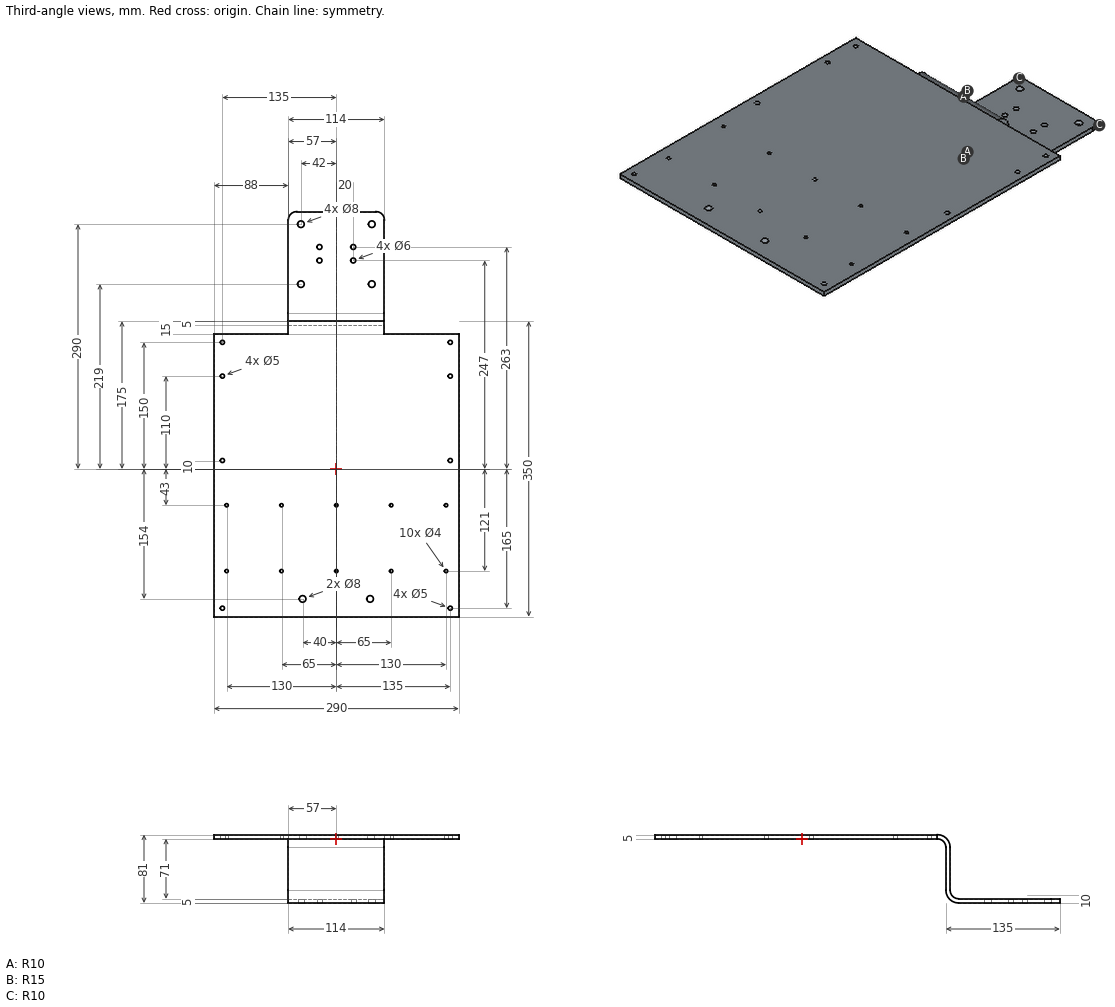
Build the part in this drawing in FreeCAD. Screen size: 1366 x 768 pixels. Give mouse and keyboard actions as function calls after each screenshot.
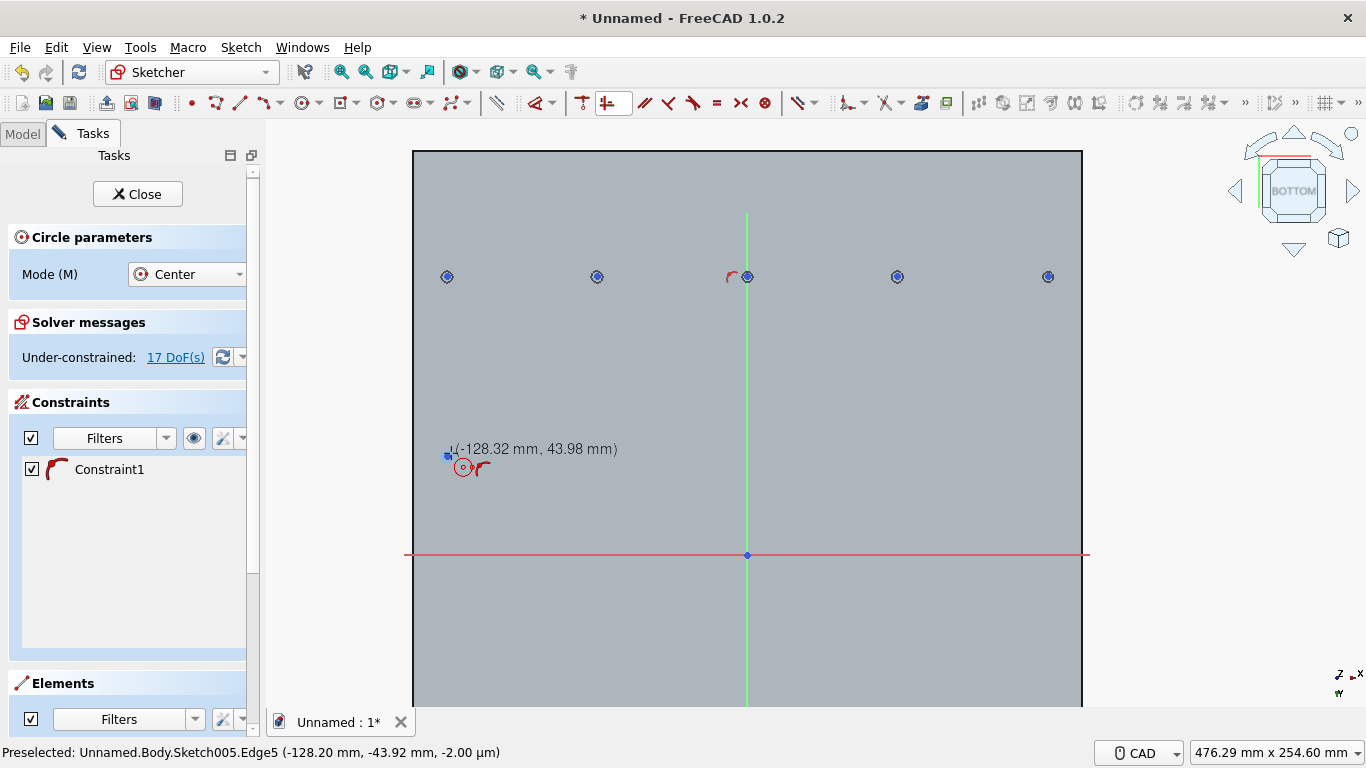
click(597, 456)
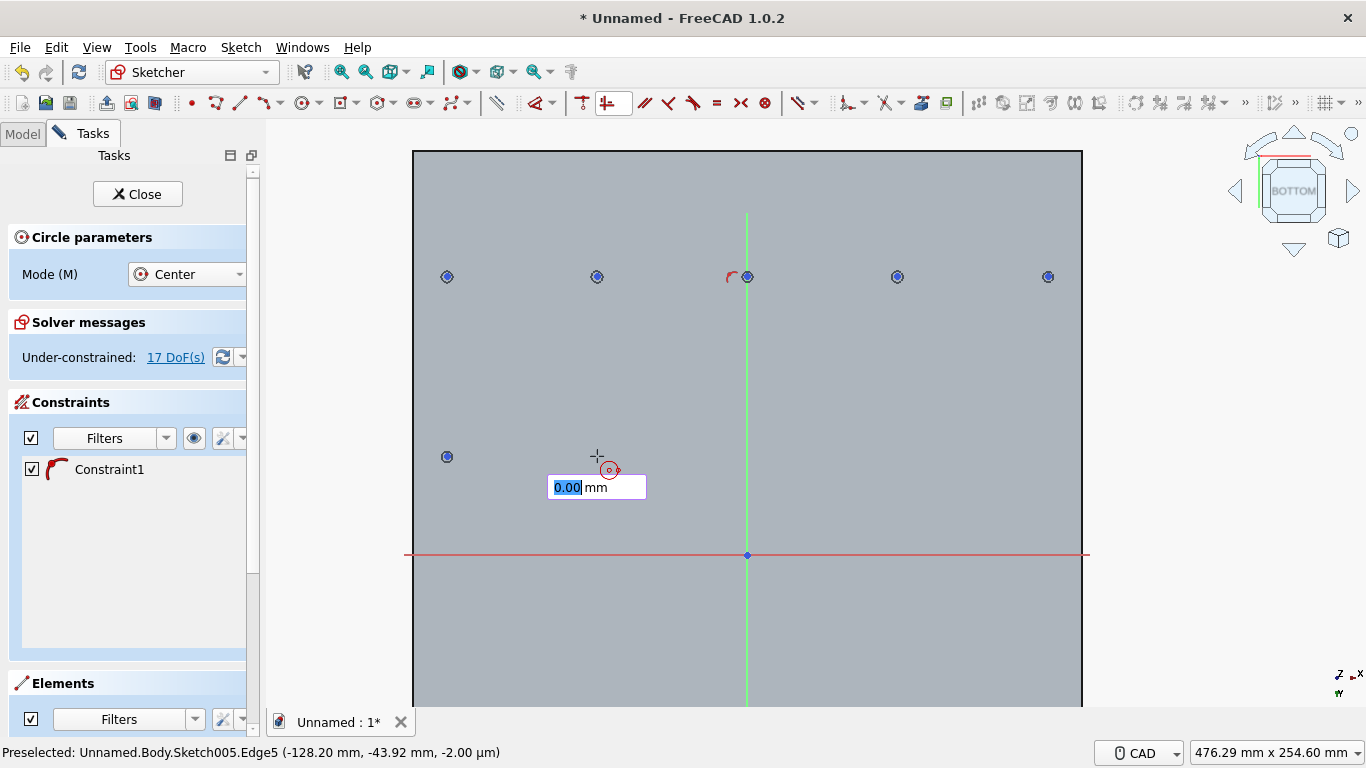
scroll(601, 453, up, 7)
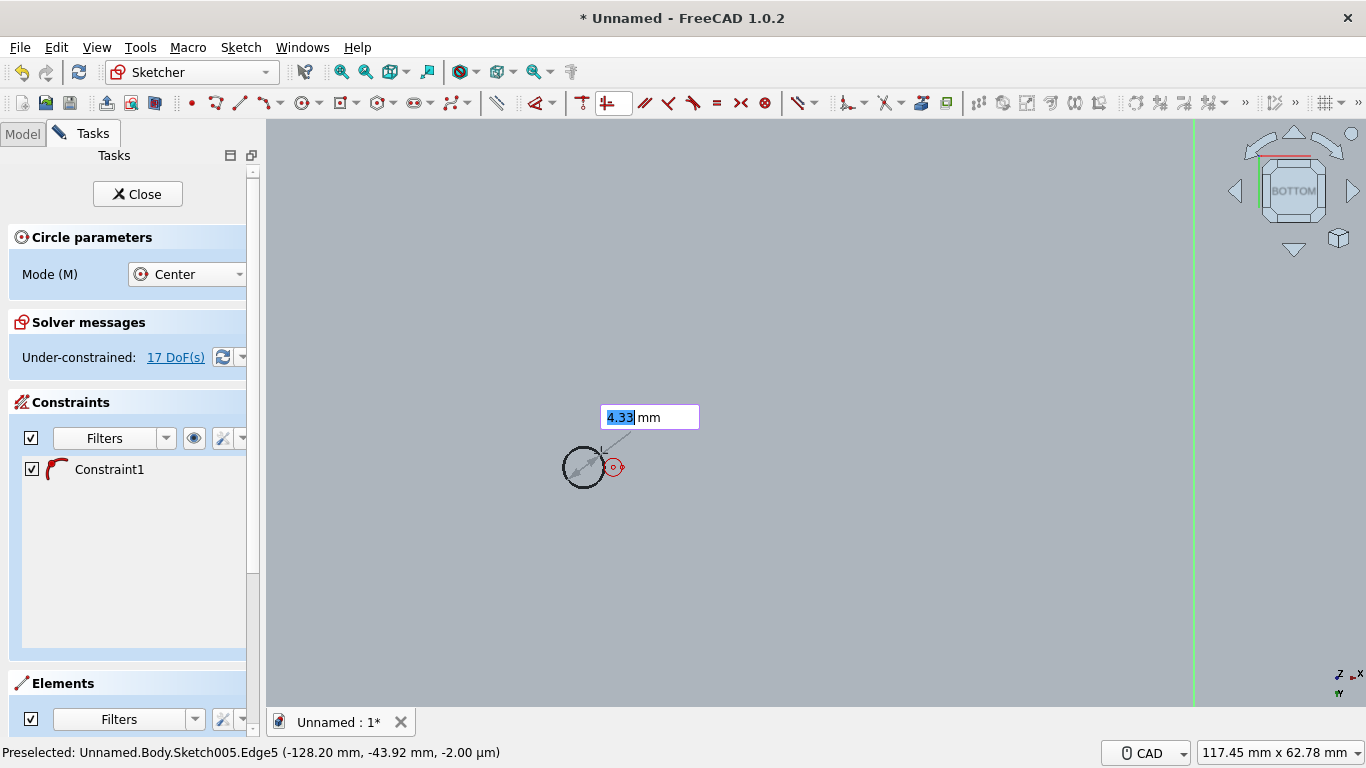
click(599, 450)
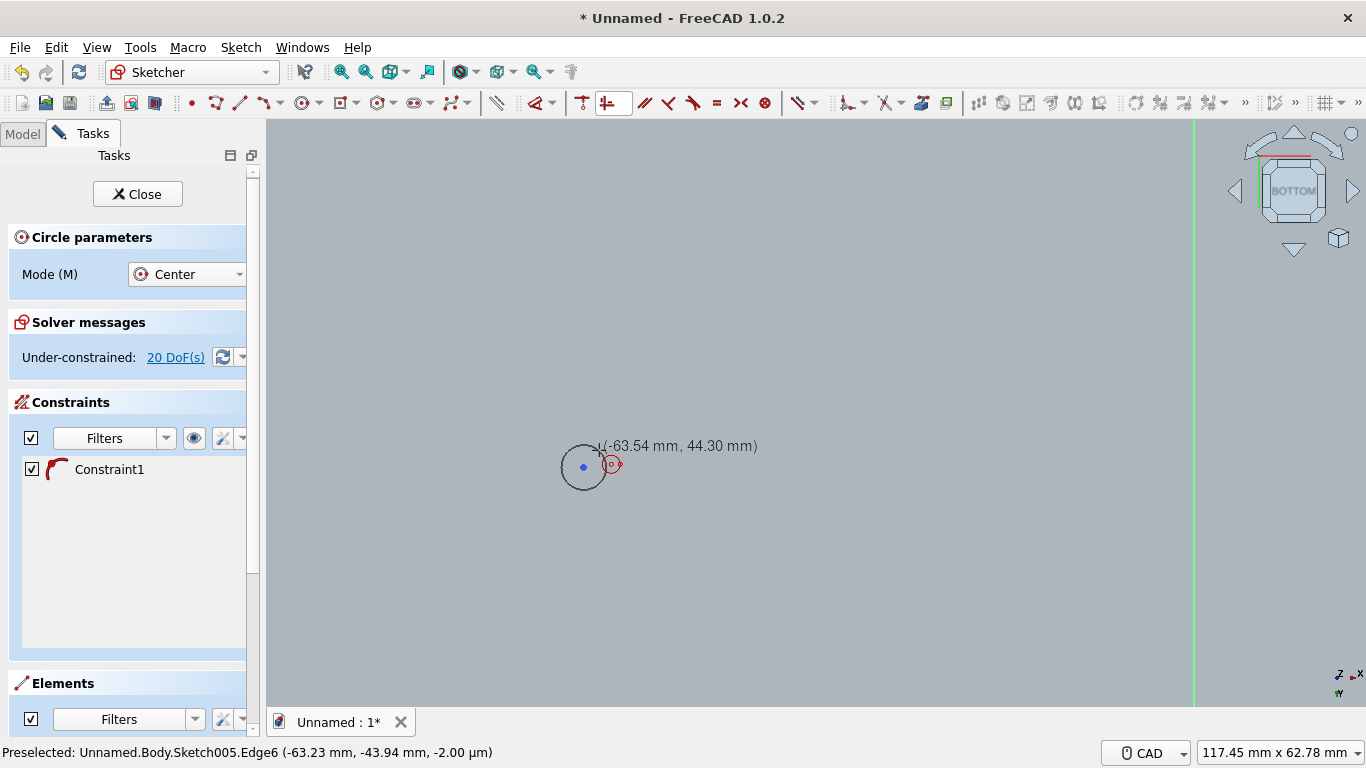
scroll(601, 453, down, 7)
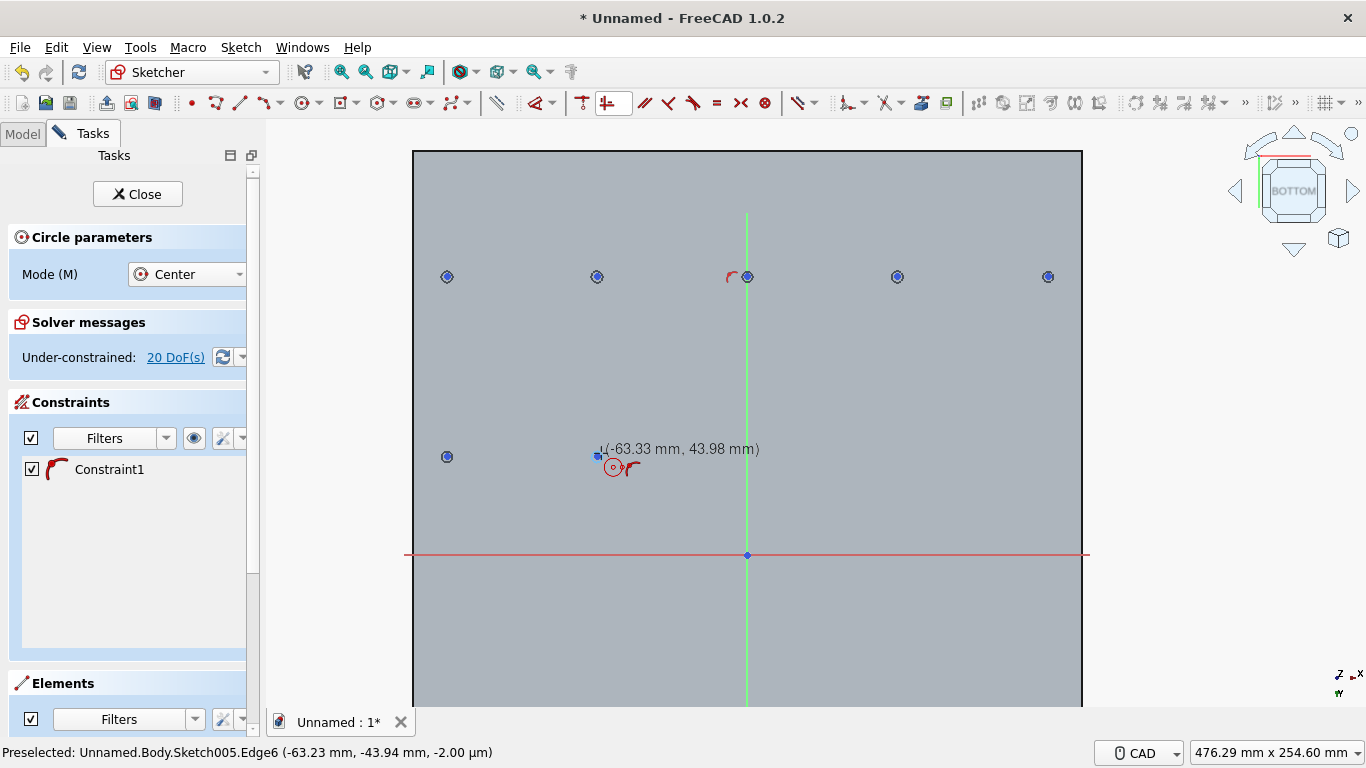
click(747, 456)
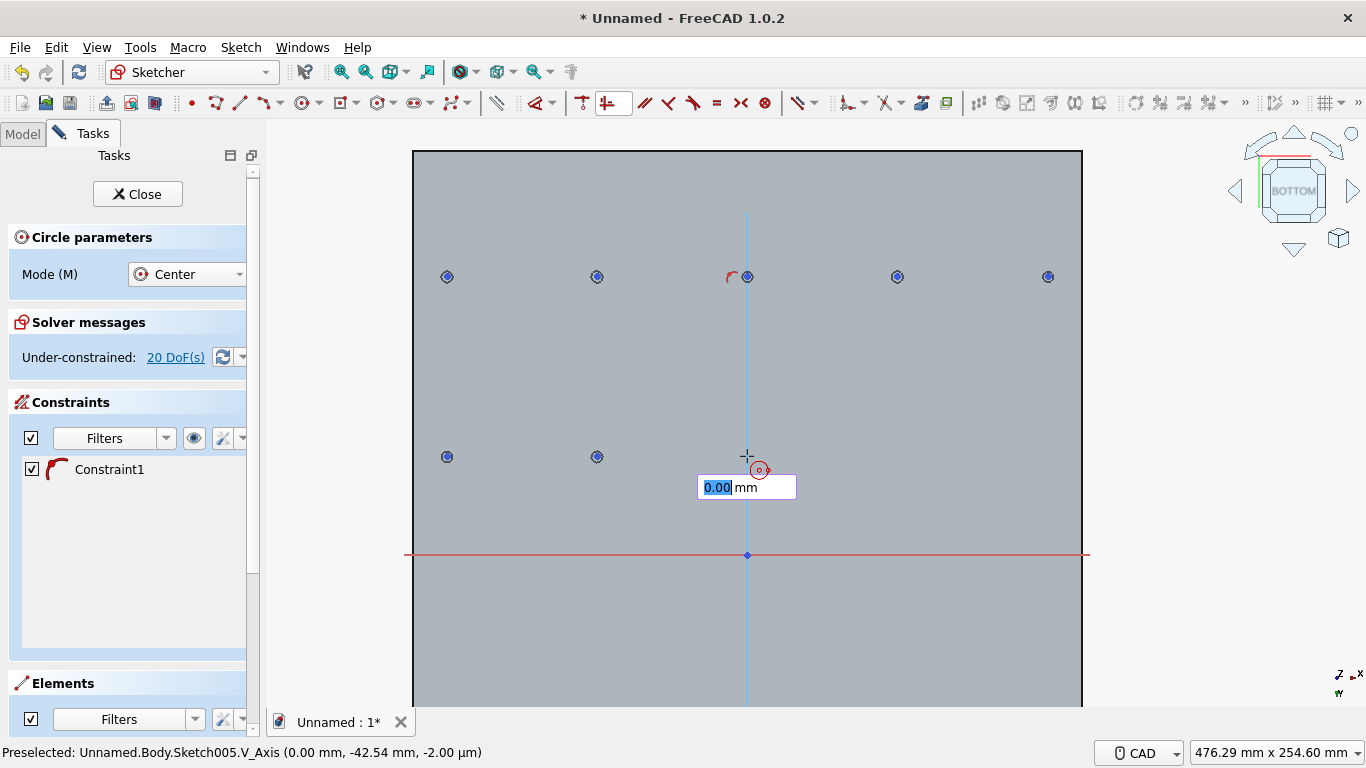
scroll(752, 454, up, 7)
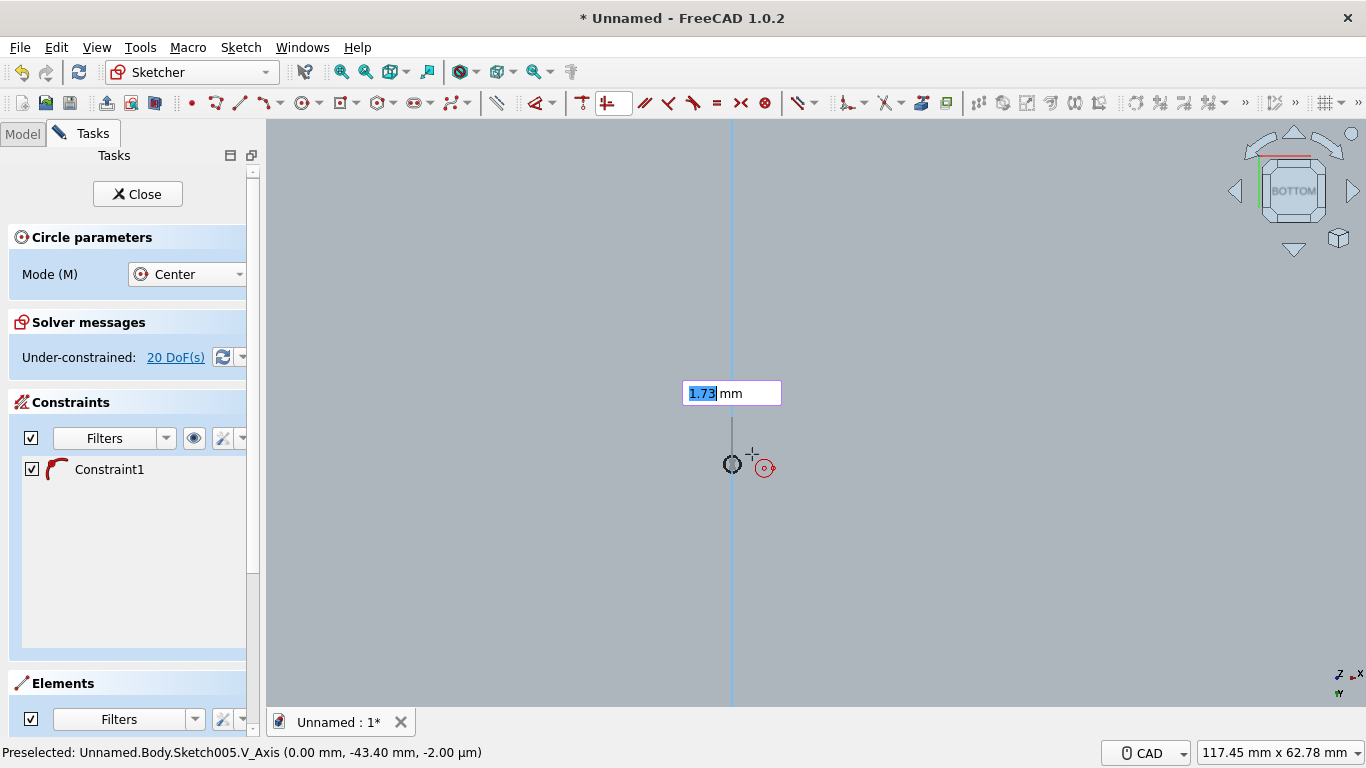
click(750, 454)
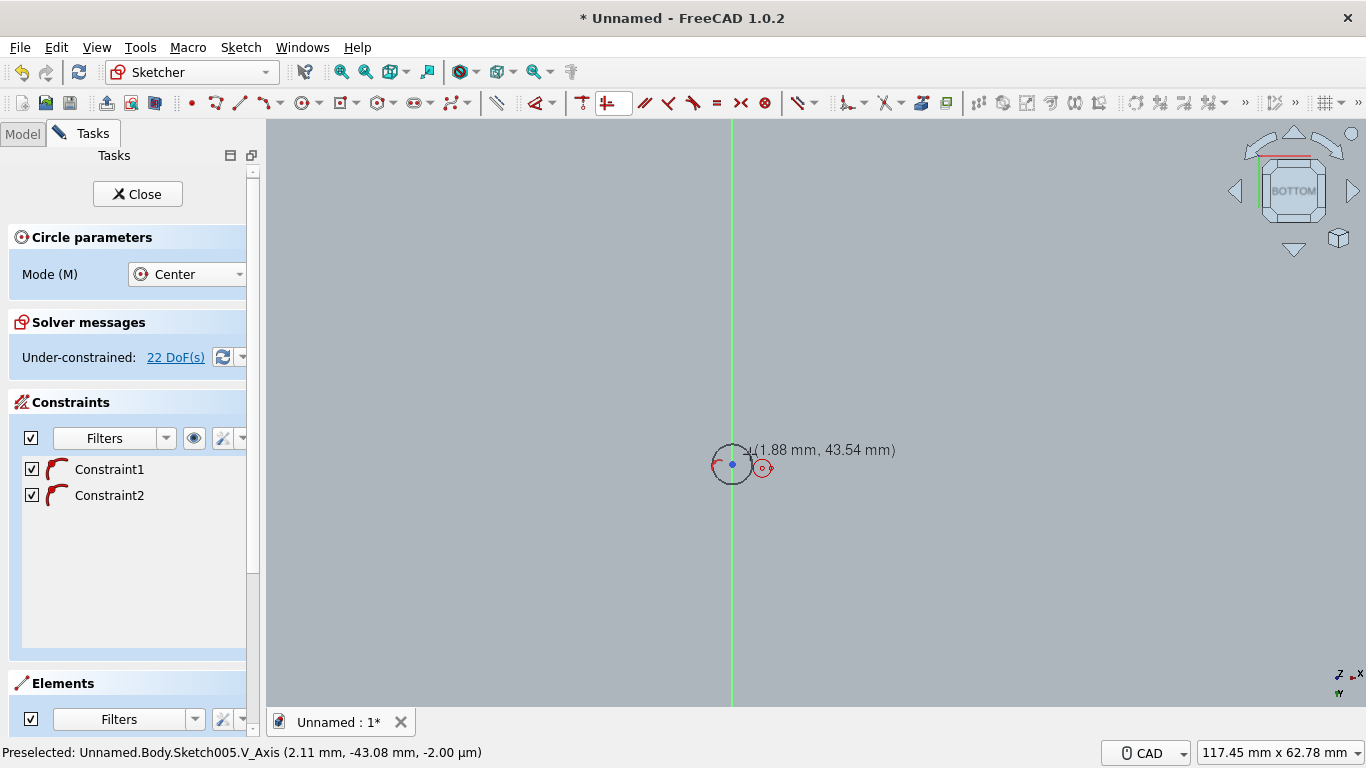
scroll(752, 454, down, 7)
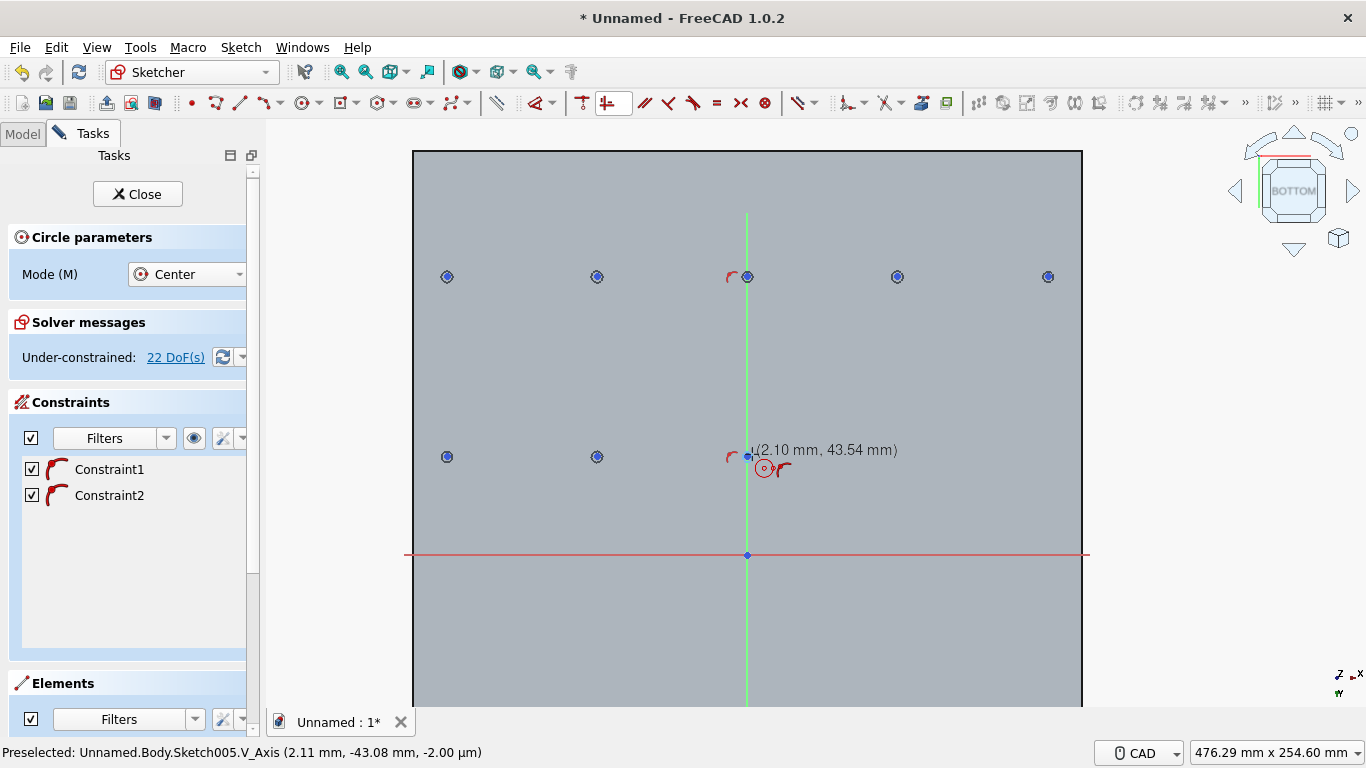
scroll(898, 456, up, 8)